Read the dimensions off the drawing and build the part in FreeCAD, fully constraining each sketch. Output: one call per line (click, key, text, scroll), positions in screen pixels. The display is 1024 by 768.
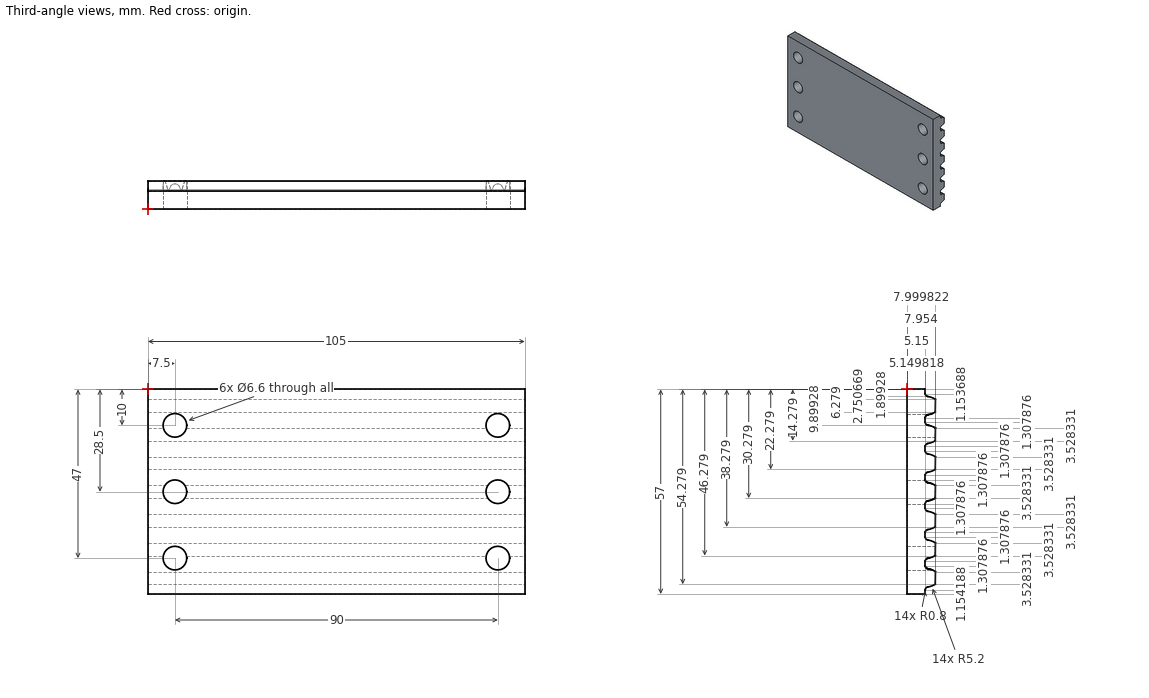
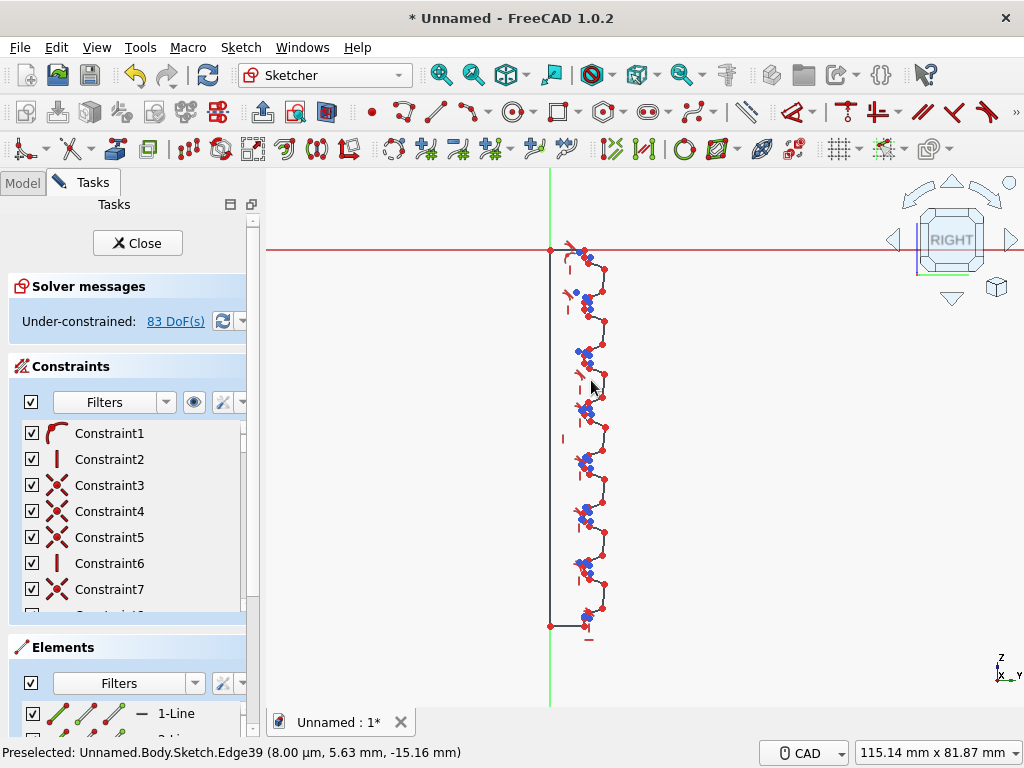
scroll(593, 349, up, 6)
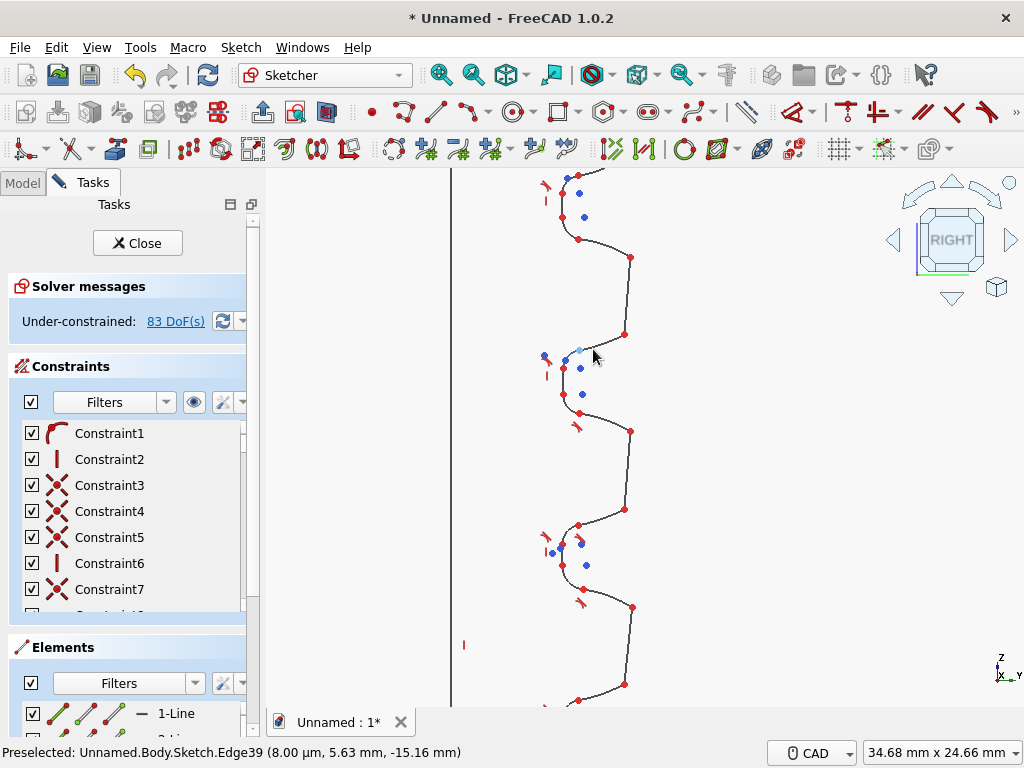
click(593, 347)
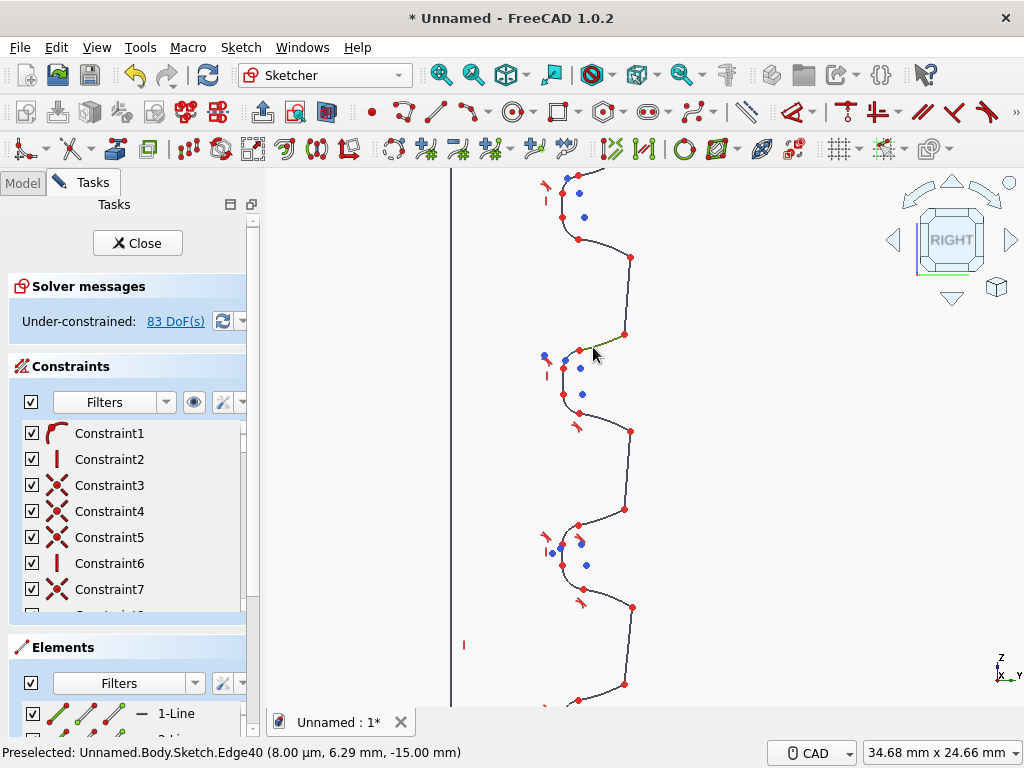
click(988, 112)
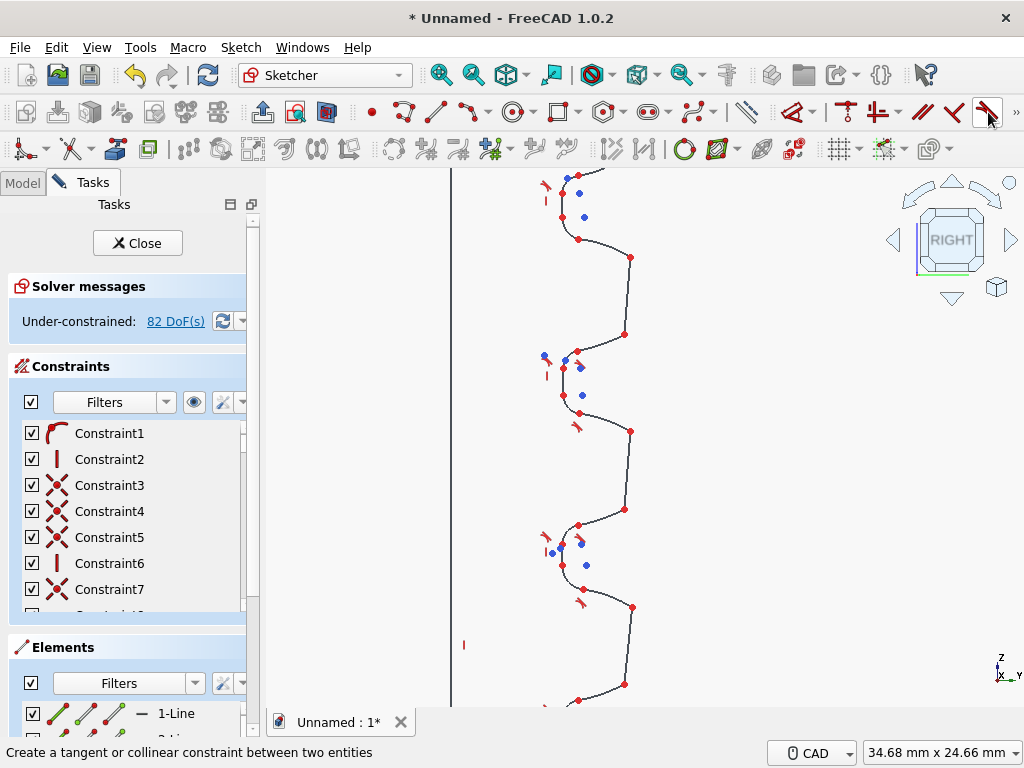
click(616, 249)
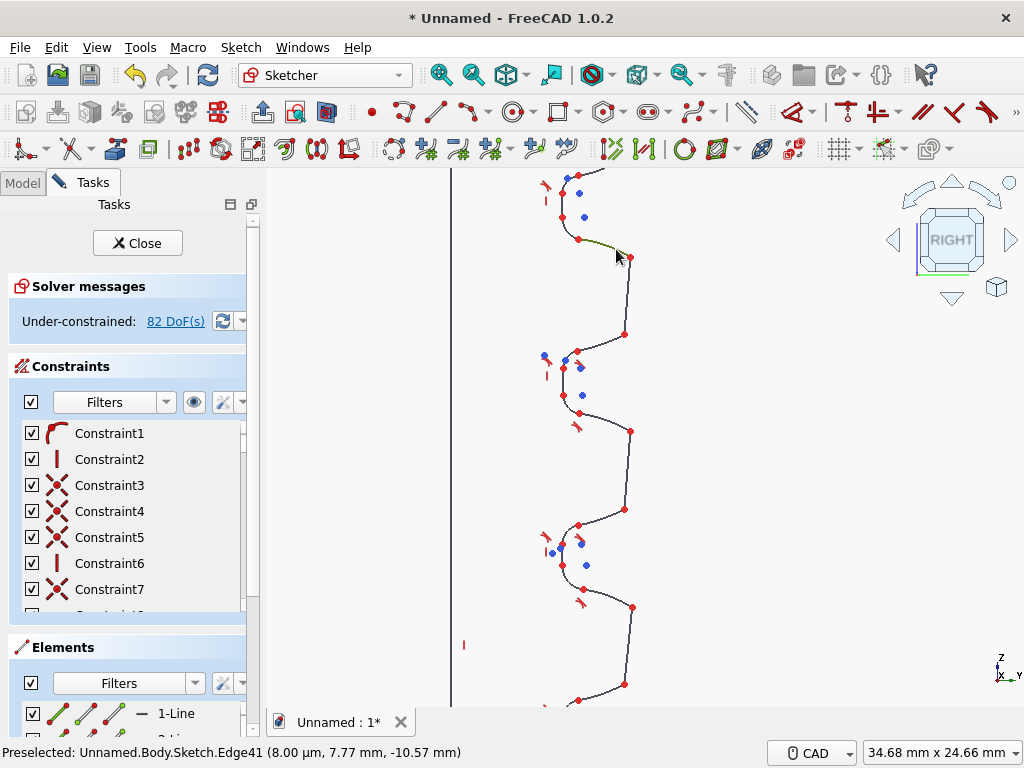
click(567, 231)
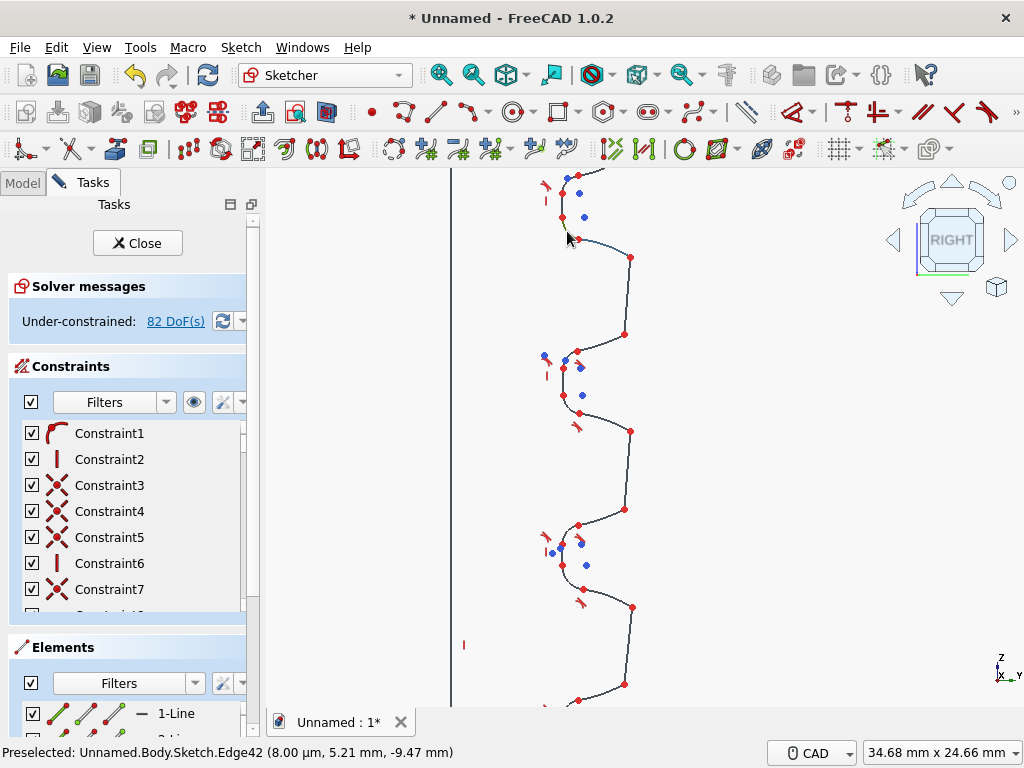
click(988, 112)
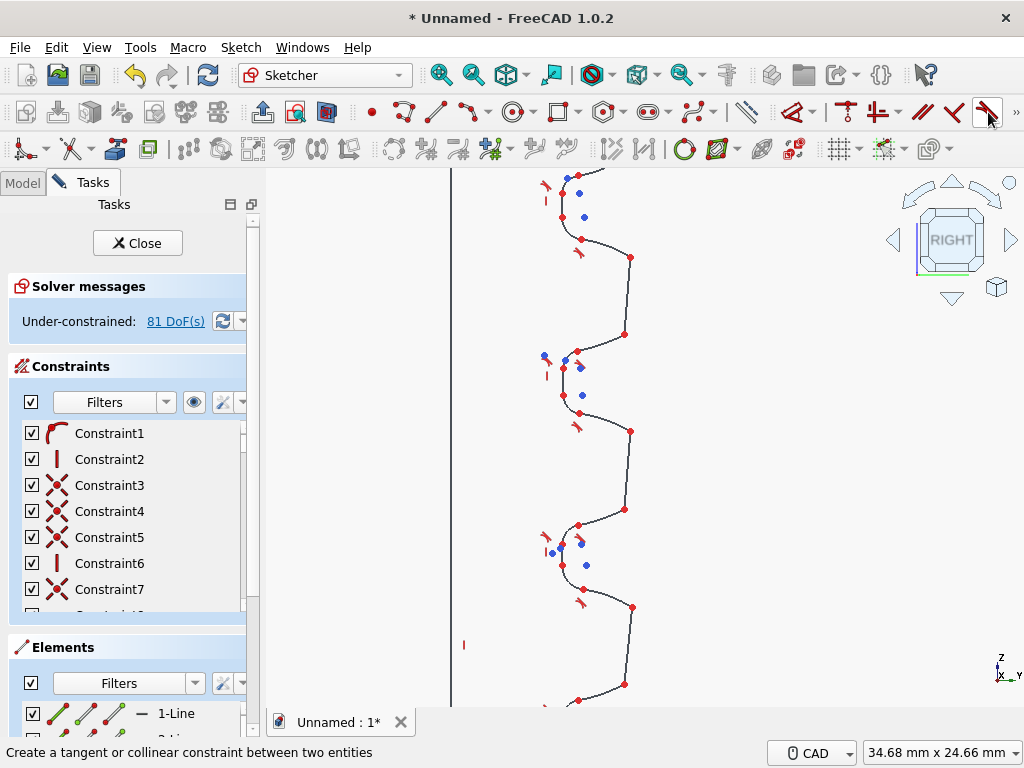
scroll(593, 349, down, 6)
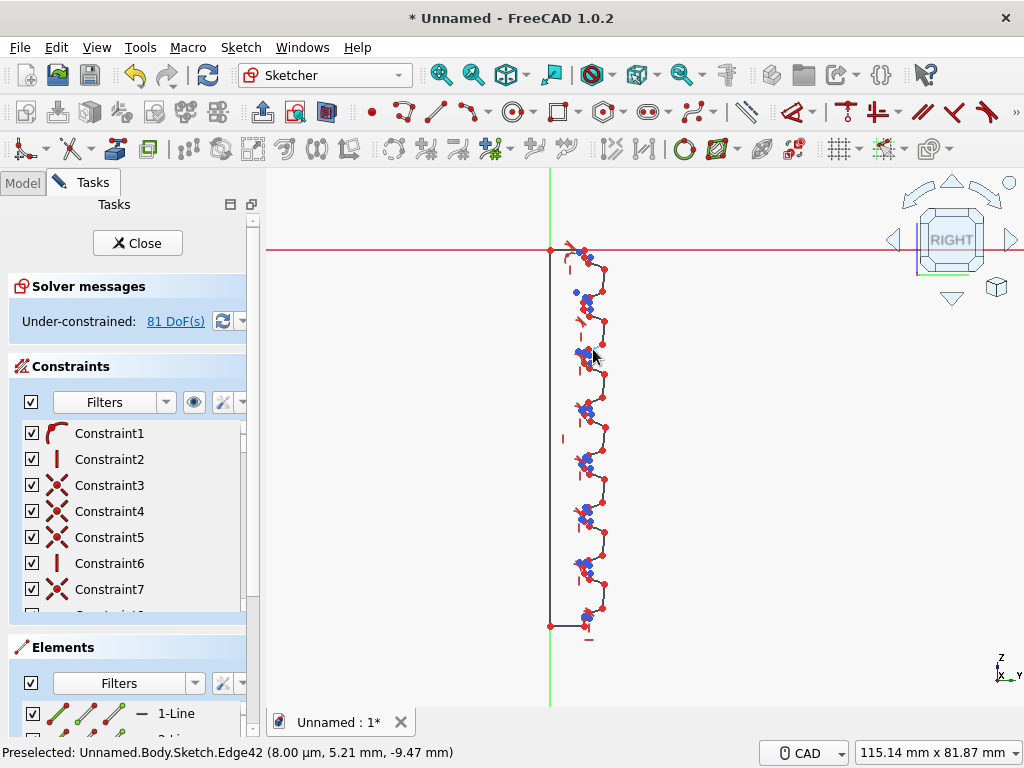
scroll(585, 299, up, 7)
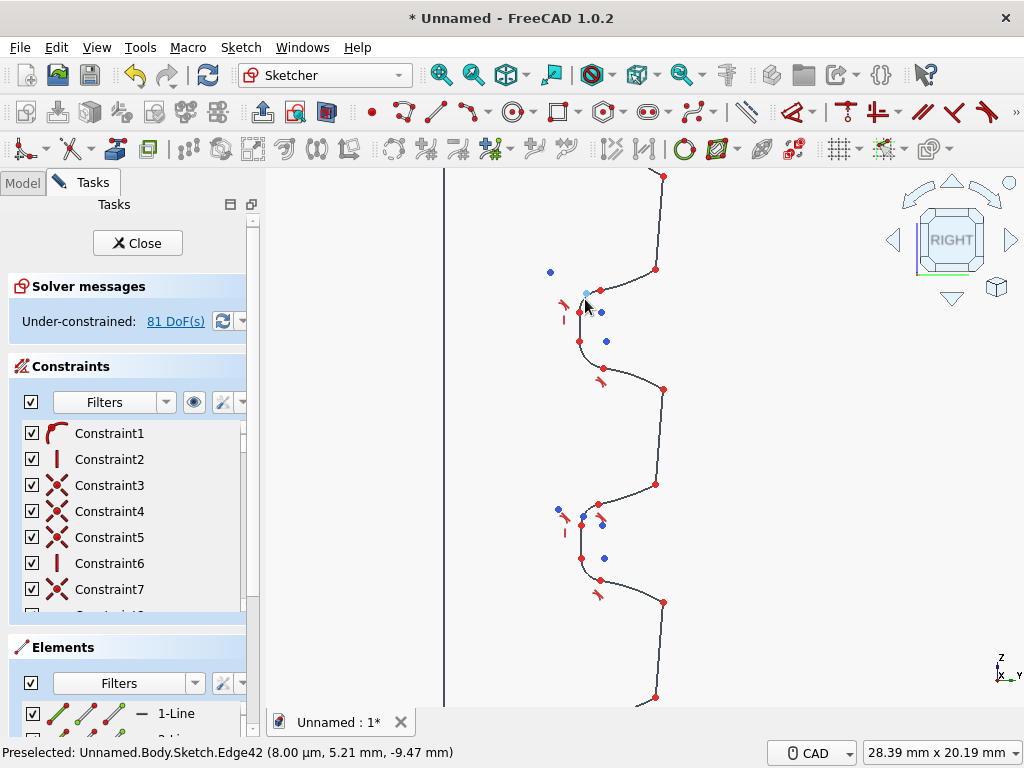
click(582, 303)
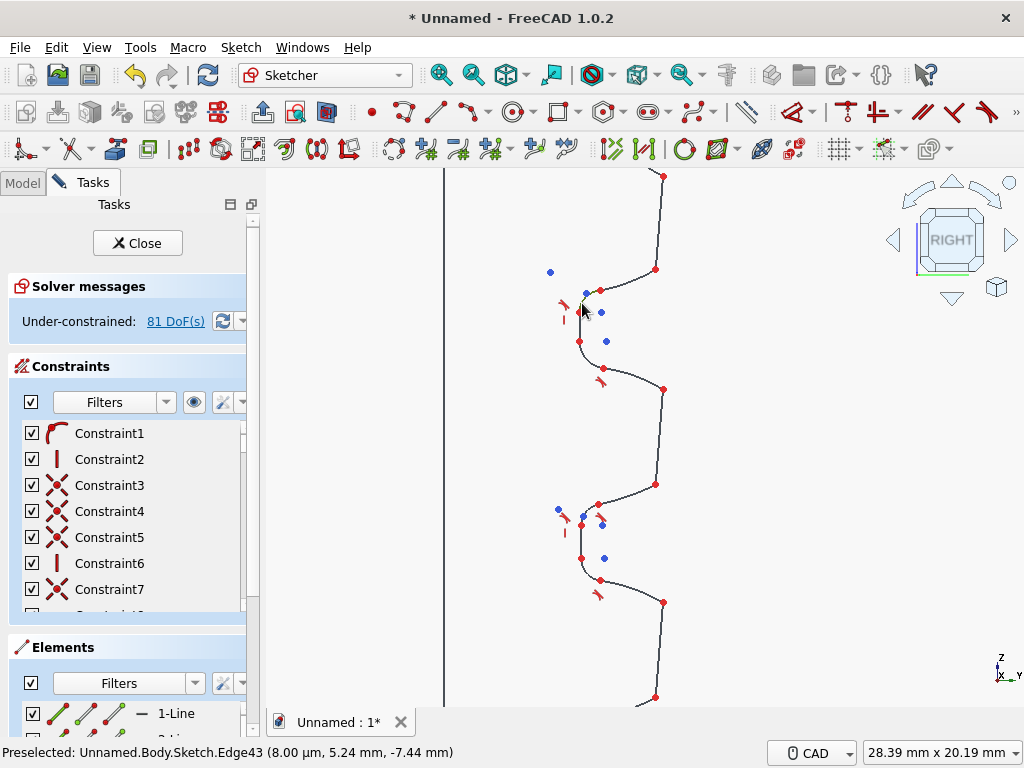
click(617, 286)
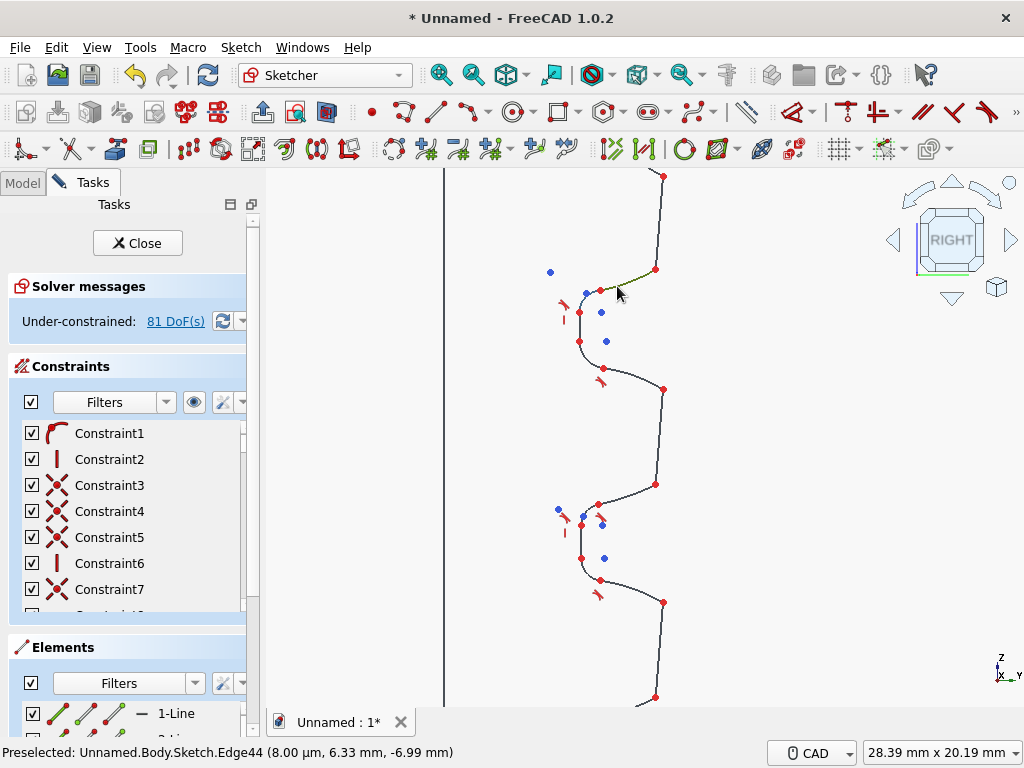
click(988, 112)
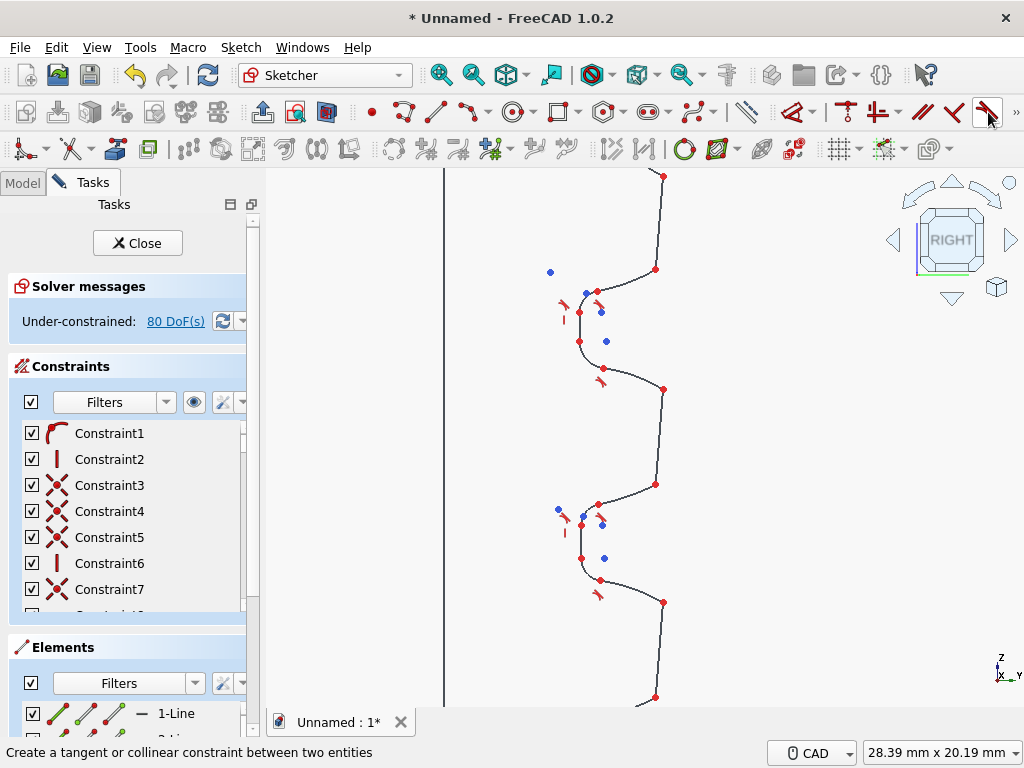
scroll(585, 299, down, 7)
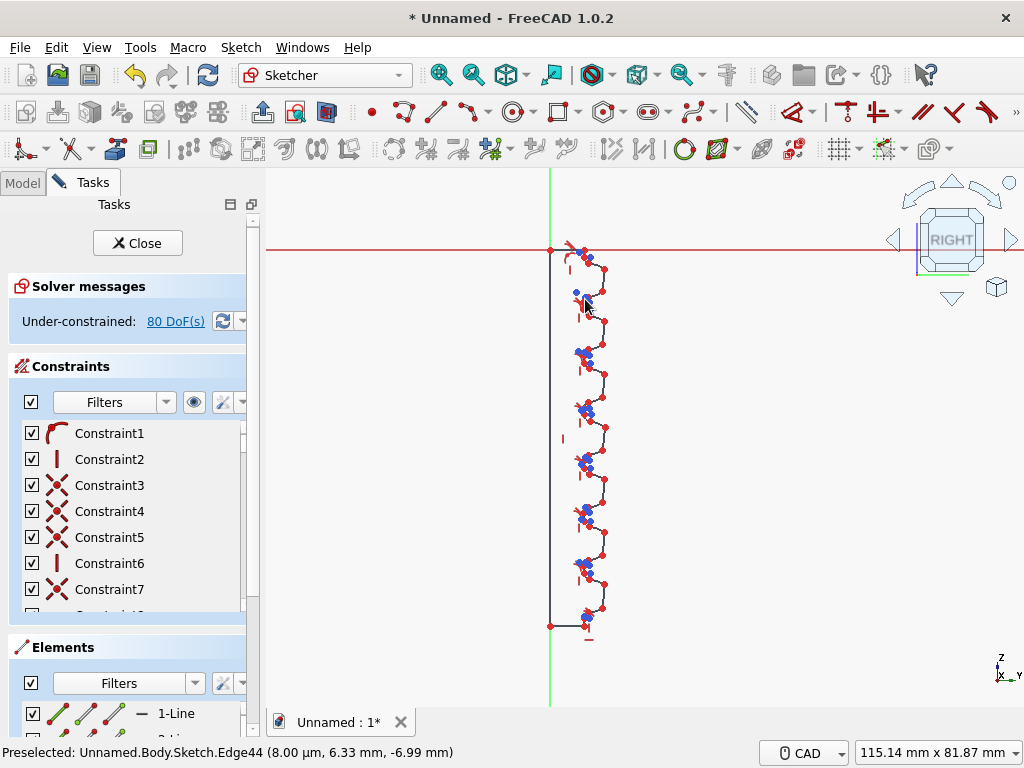
scroll(600, 267, up, 6)